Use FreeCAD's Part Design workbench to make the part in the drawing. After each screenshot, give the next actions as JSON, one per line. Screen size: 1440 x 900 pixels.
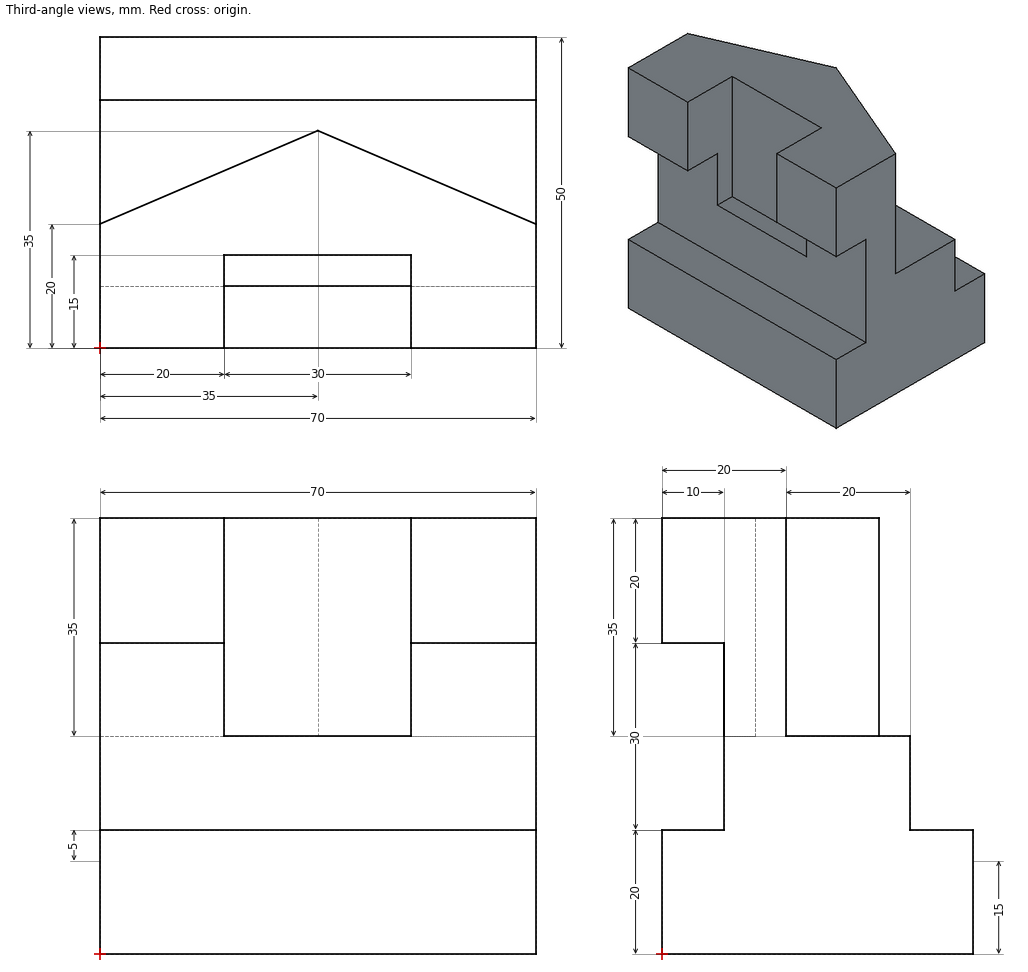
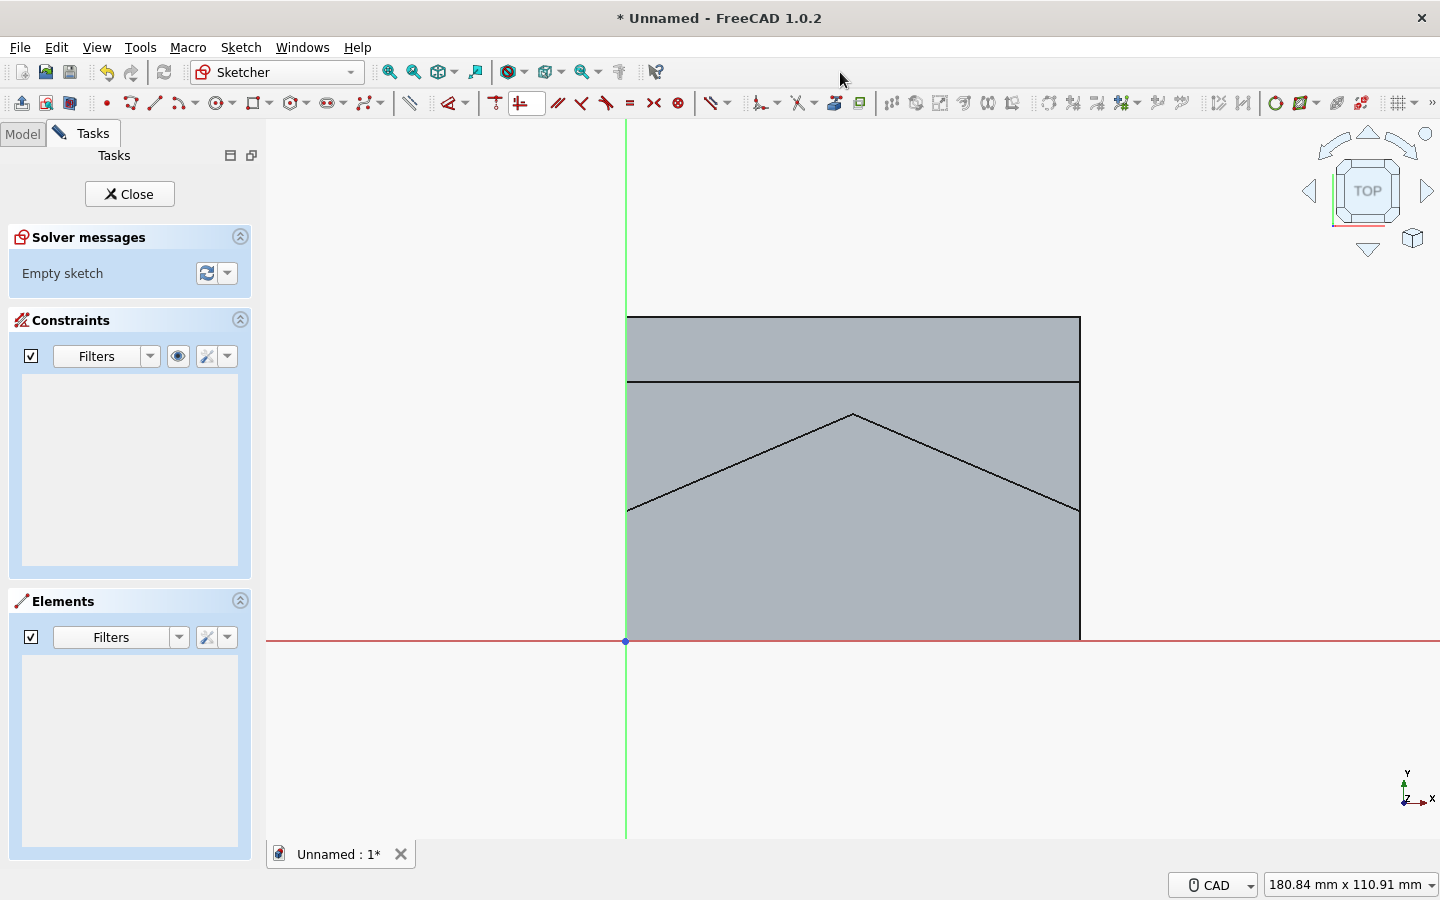
{"action": "scroll", "coordinate": [791, 685], "scroll_direction": "up", "scroll_amount": 4}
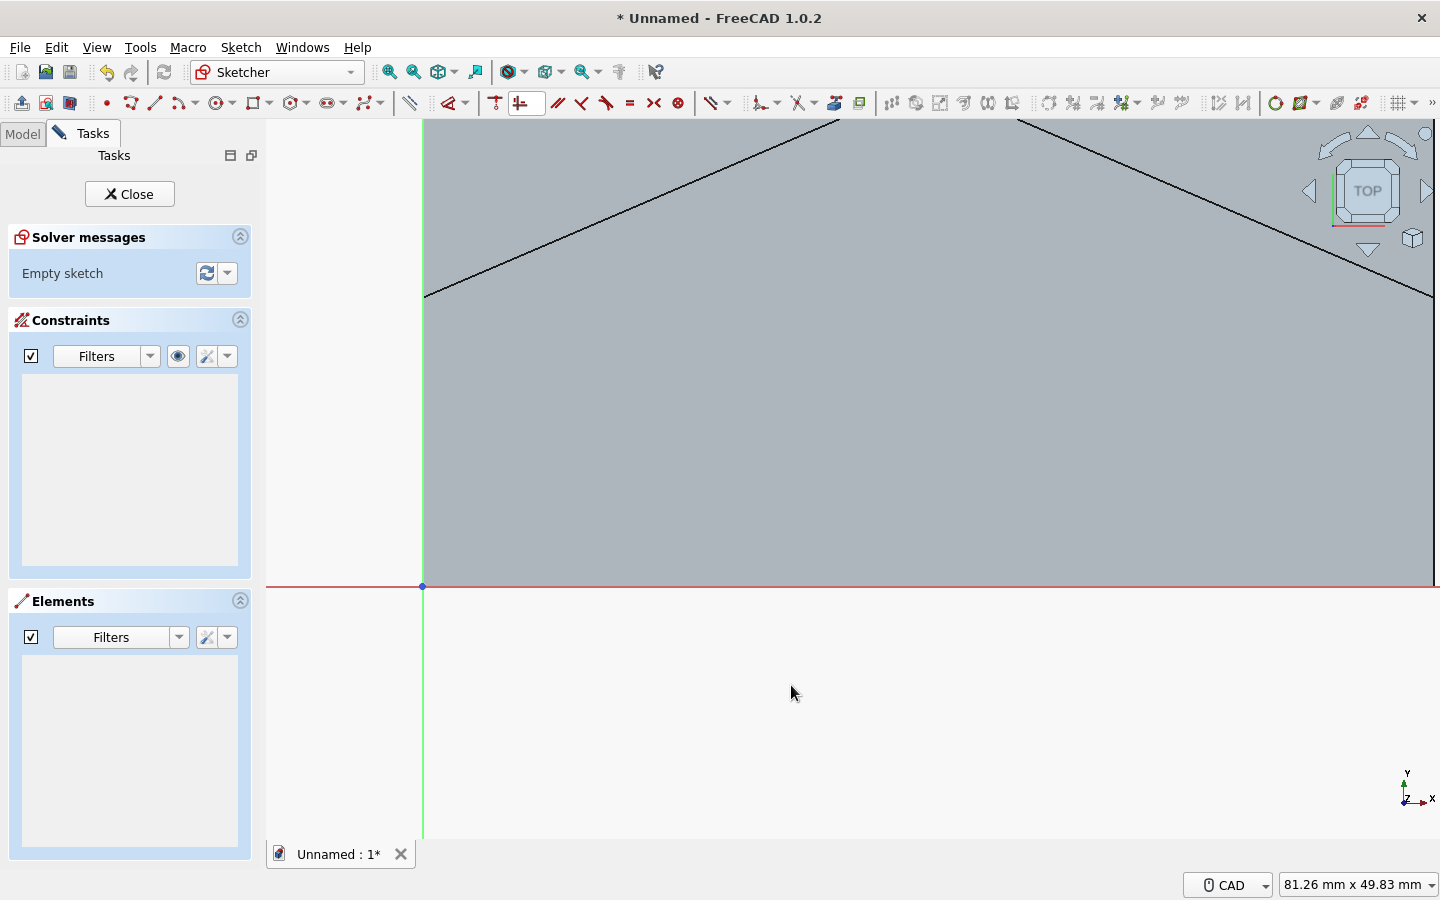
{"action": "left_click", "coordinate": [254, 104]}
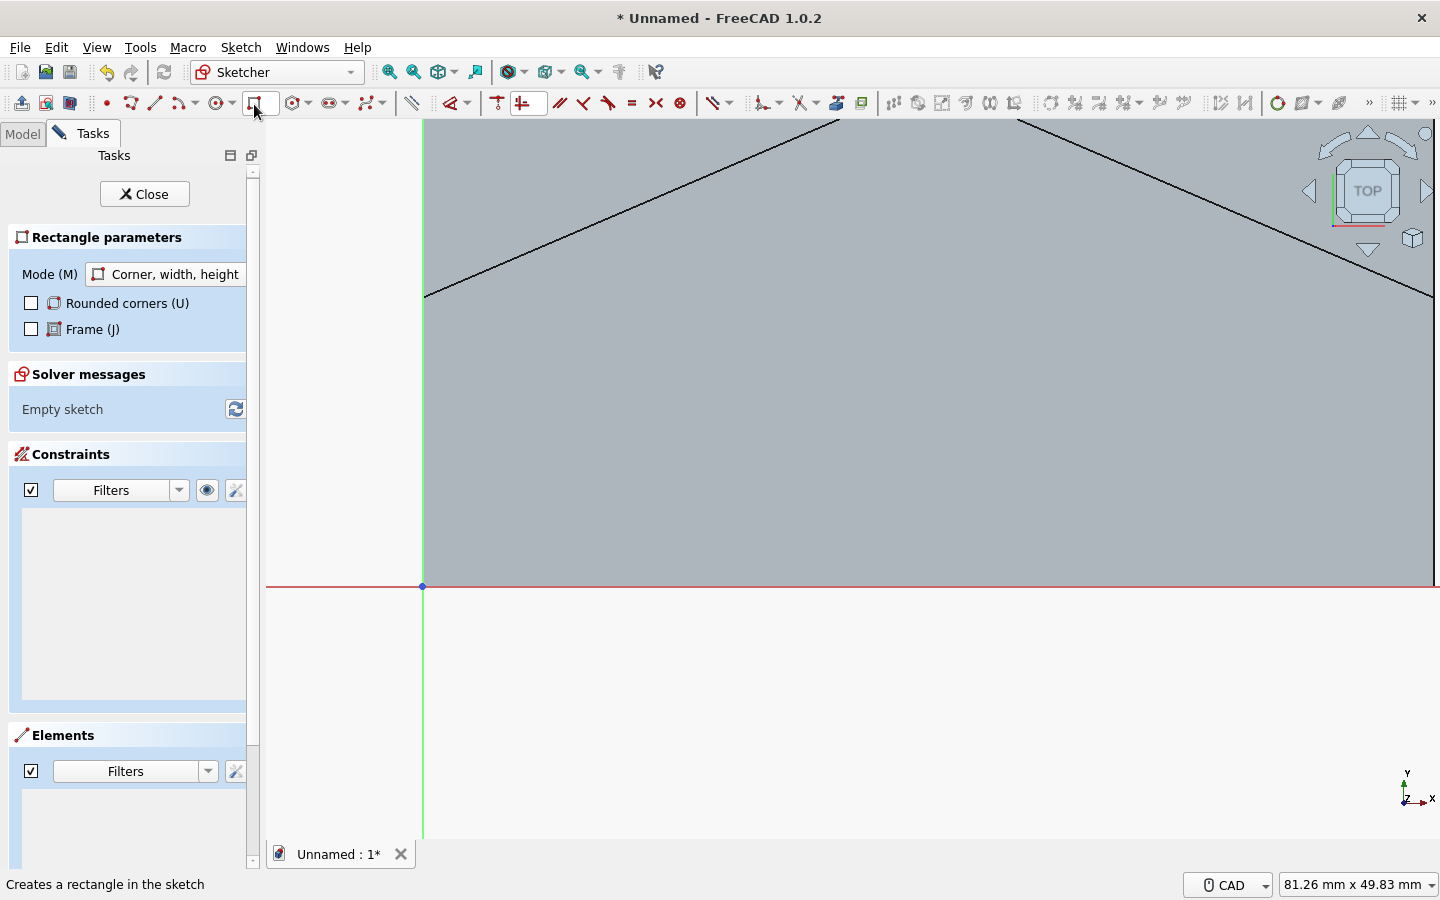
{"action": "left_click", "coordinate": [712, 370]}
{"action": "left_click", "coordinate": [1145, 587]}
{"action": "key", "text": "Escape"}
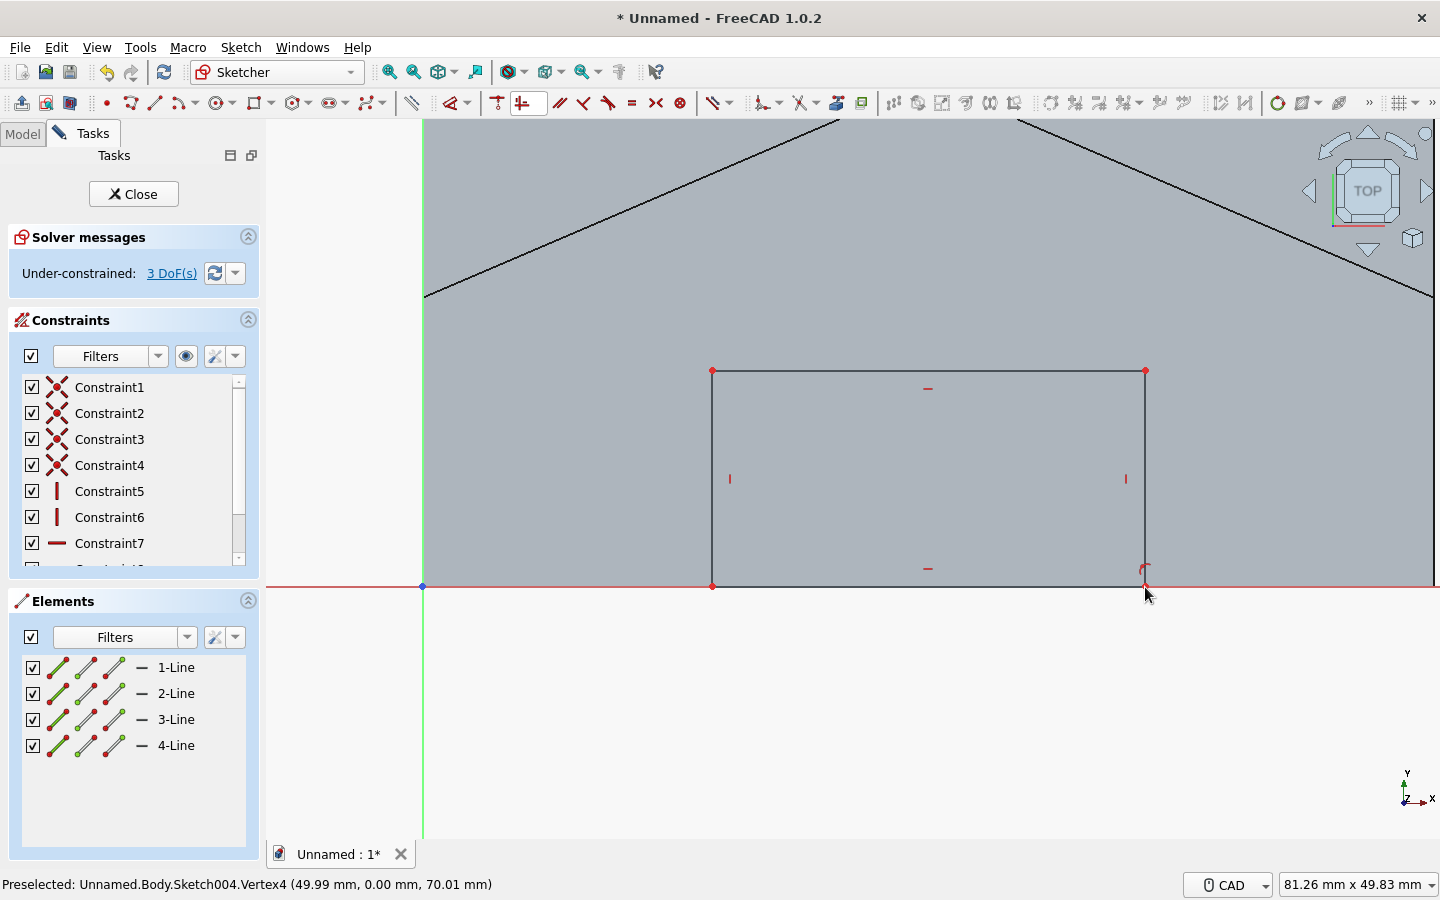
{"action": "left_click", "coordinate": [450, 104]}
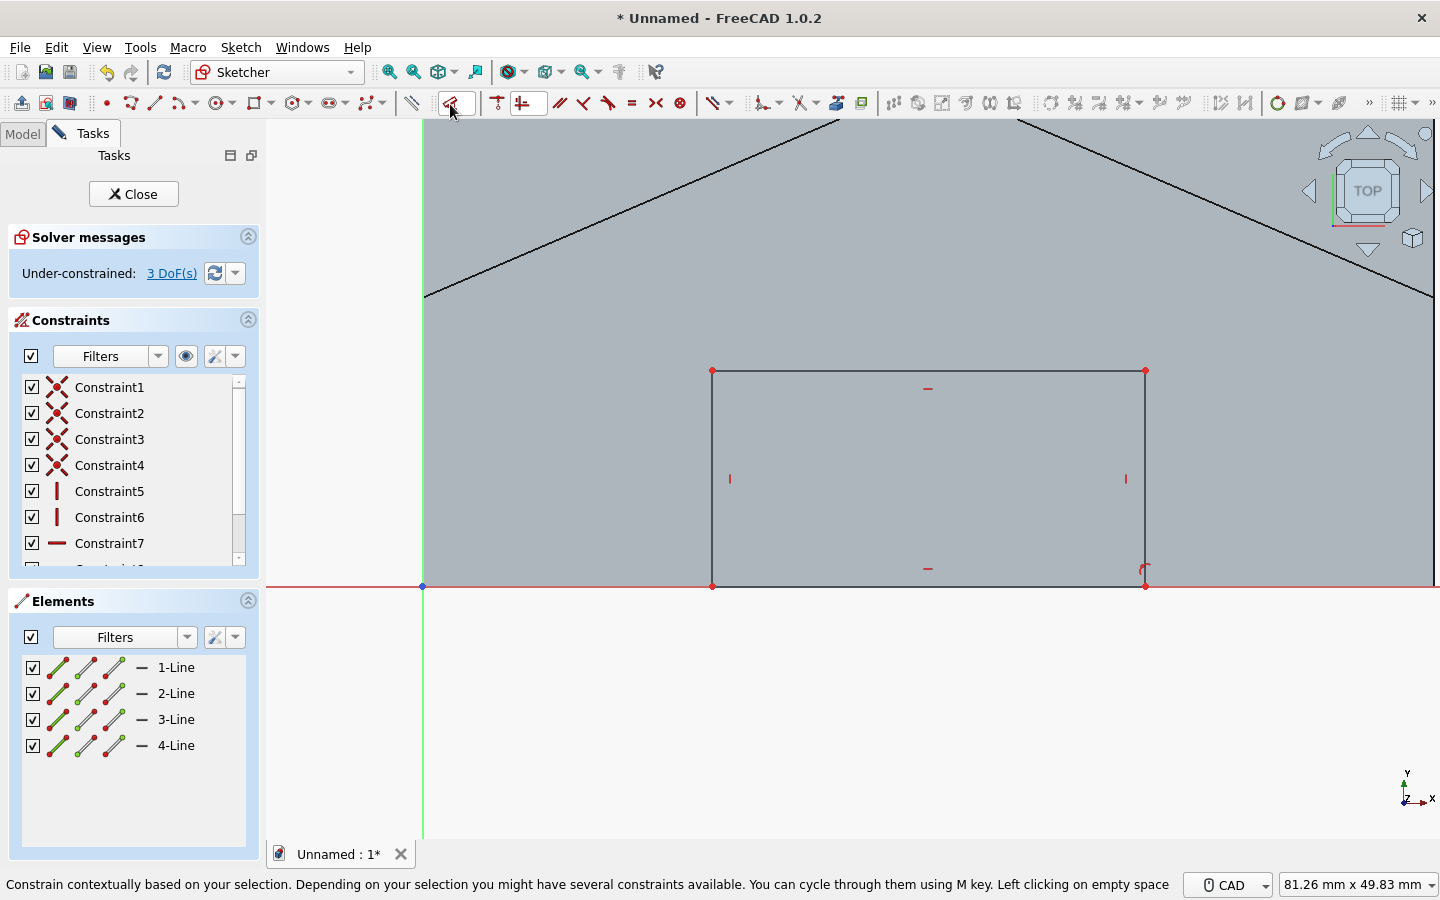
{"action": "left_click", "coordinate": [712, 436]}
{"action": "left_click", "coordinate": [678, 479]}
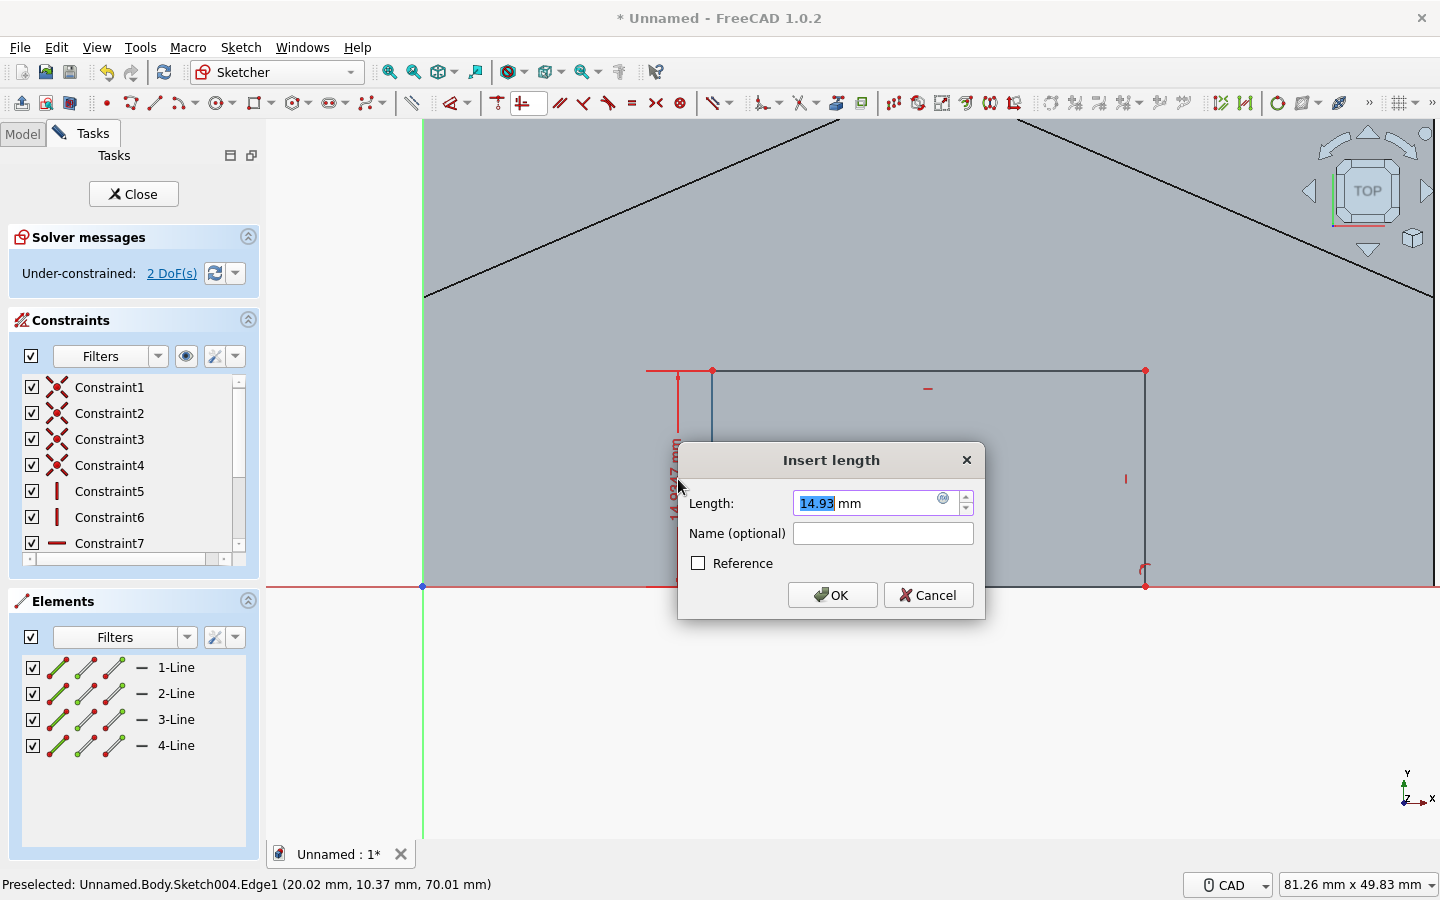
{"action": "type", "text": "15"}
{"action": "key", "text": "Return"}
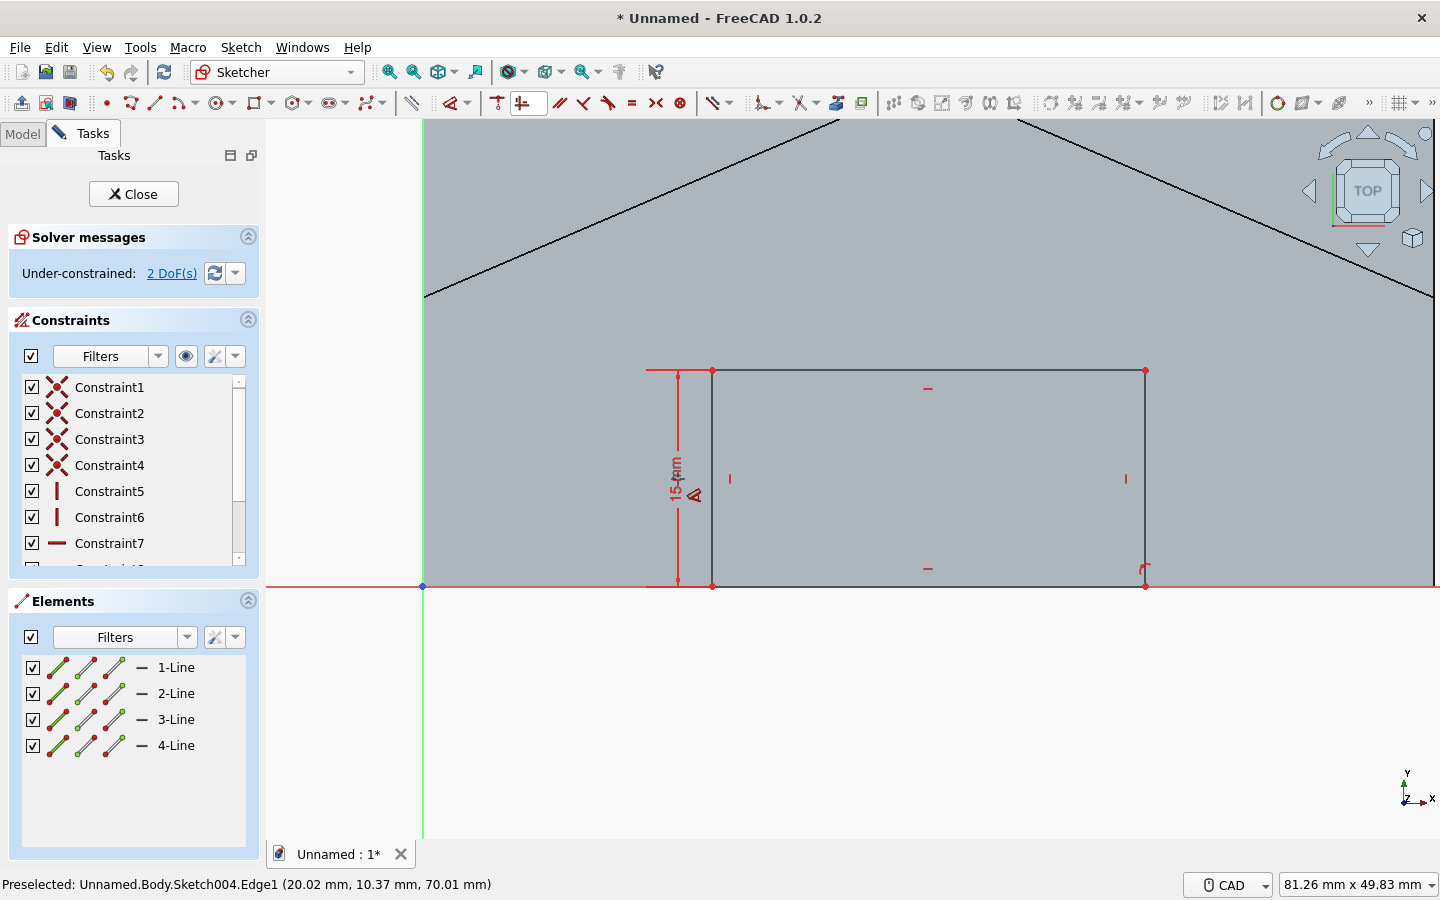
{"action": "left_click", "coordinate": [842, 587]}
{"action": "left_click", "coordinate": [929, 621]}